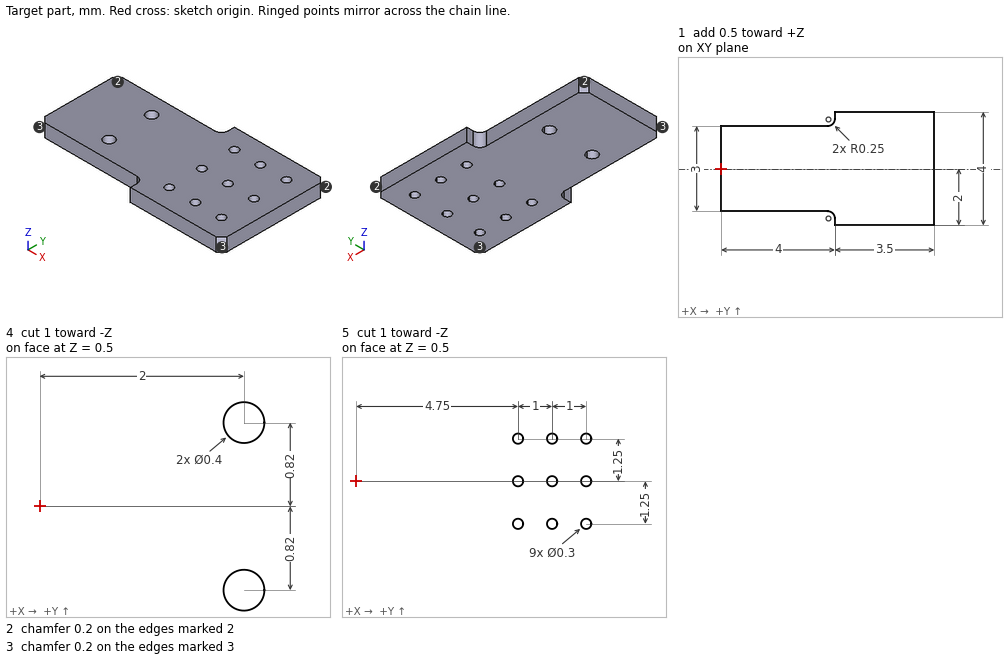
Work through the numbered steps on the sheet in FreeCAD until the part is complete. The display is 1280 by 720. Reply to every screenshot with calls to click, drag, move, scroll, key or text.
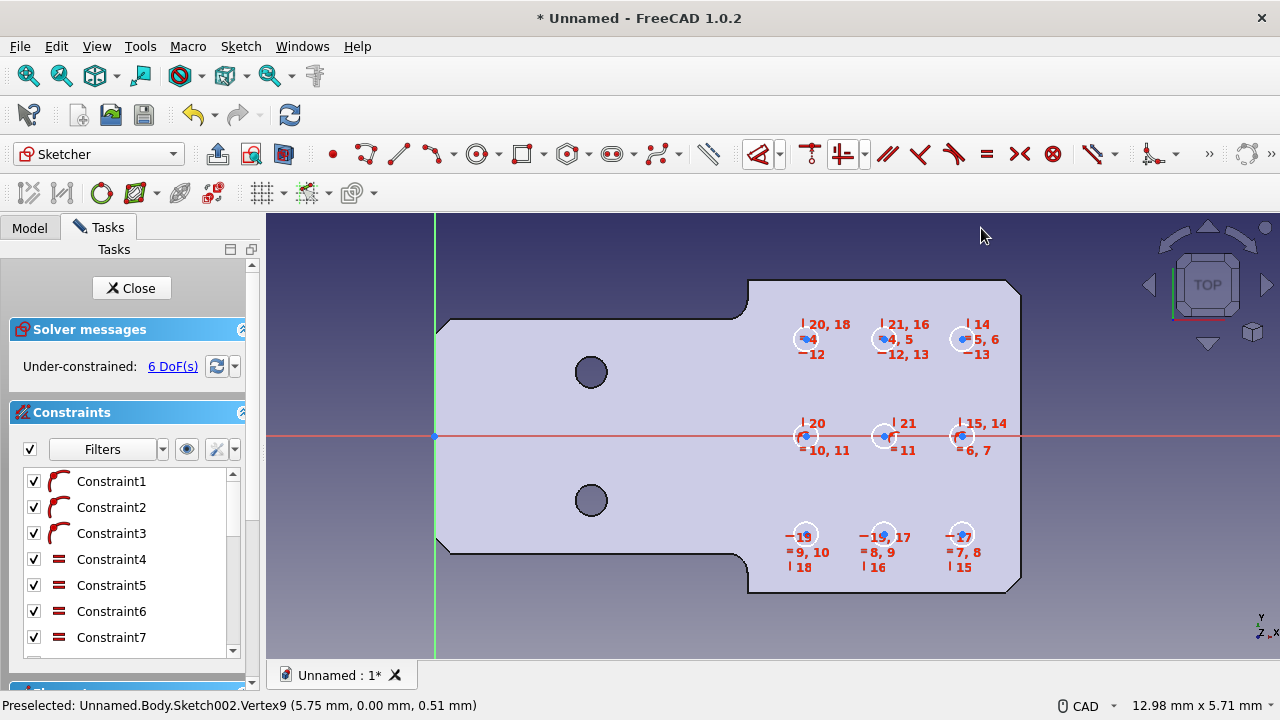
key(d)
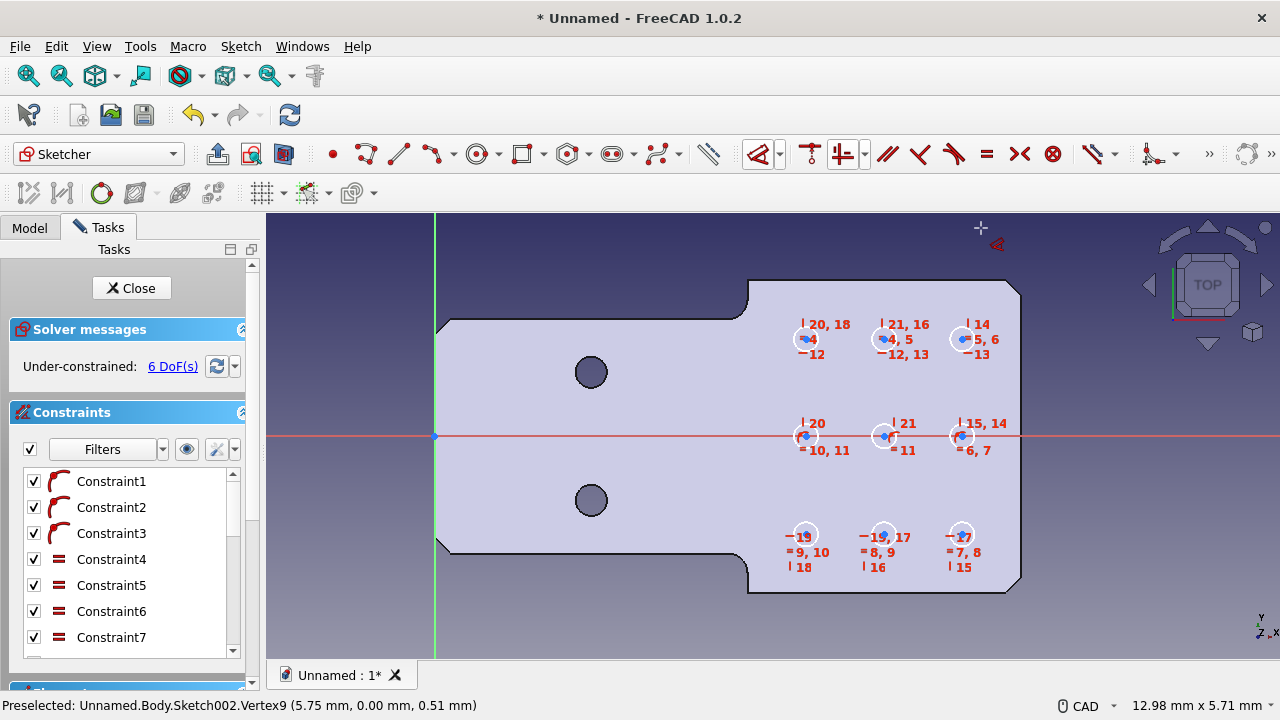
scroll(815, 331, up, 3)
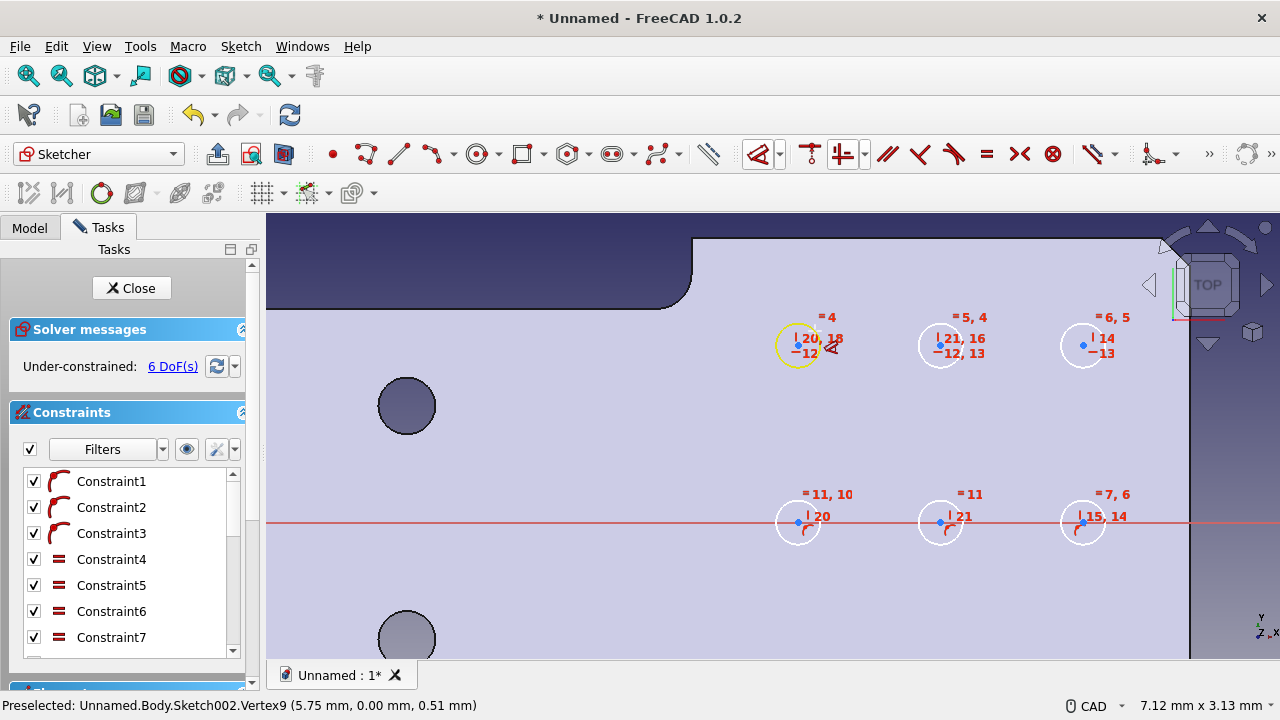
click(814, 330)
click(837, 308)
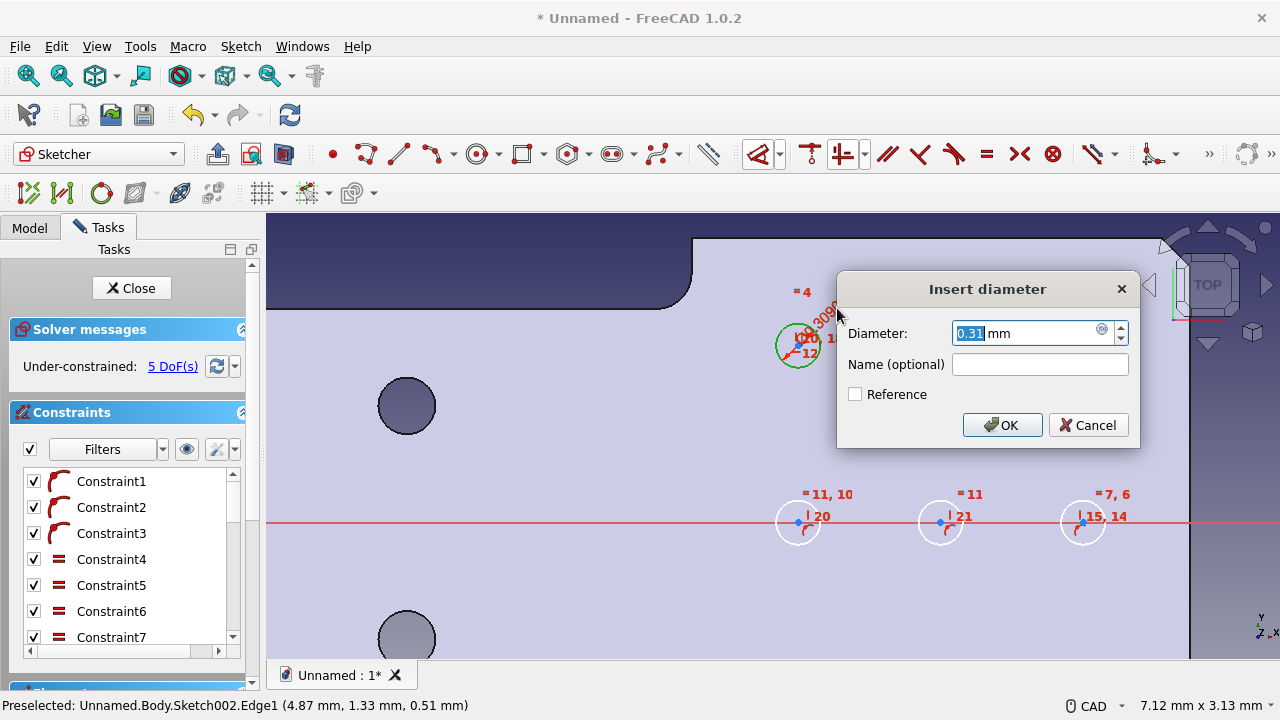
text(0.3)
key(Return)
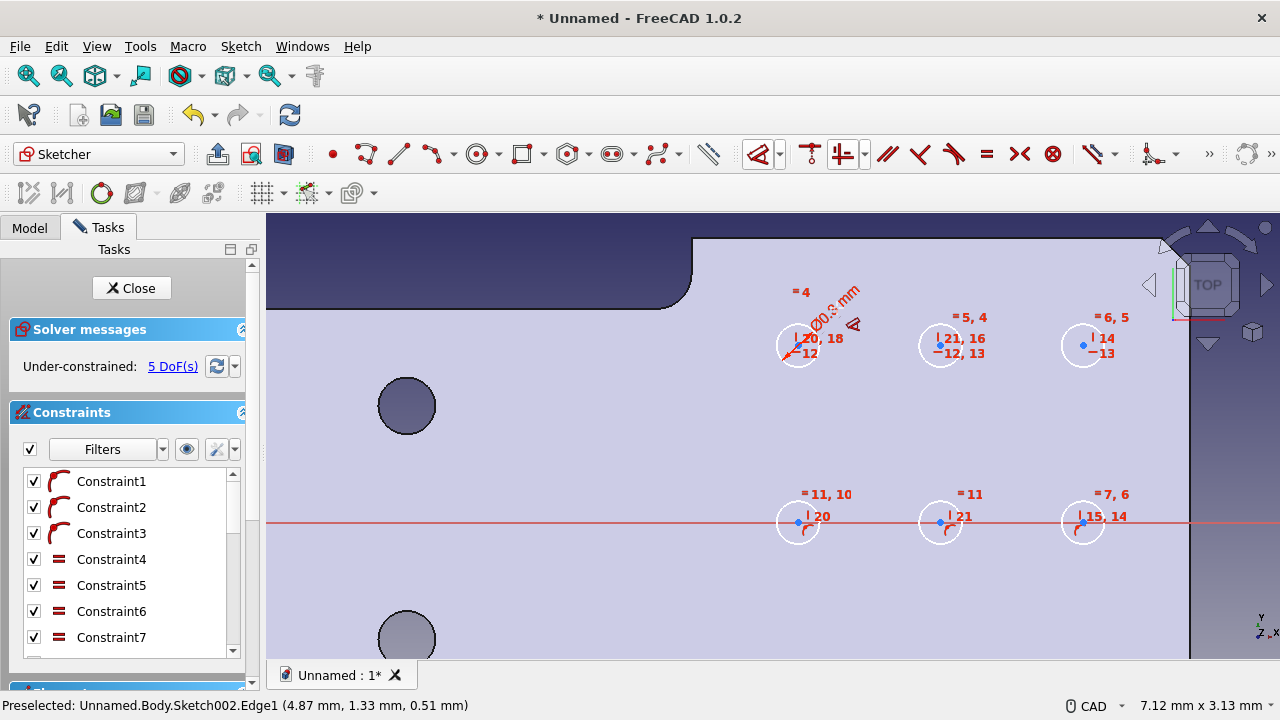
click(798, 346)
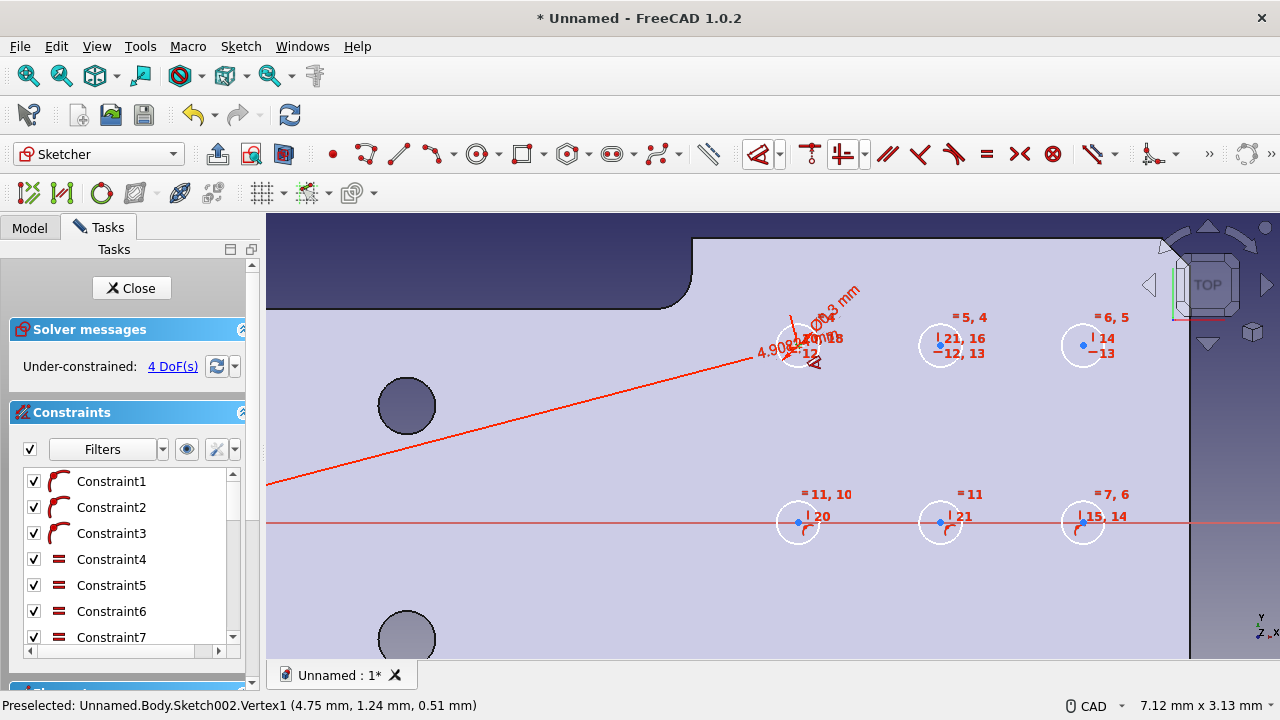
click(941, 346)
click(919, 312)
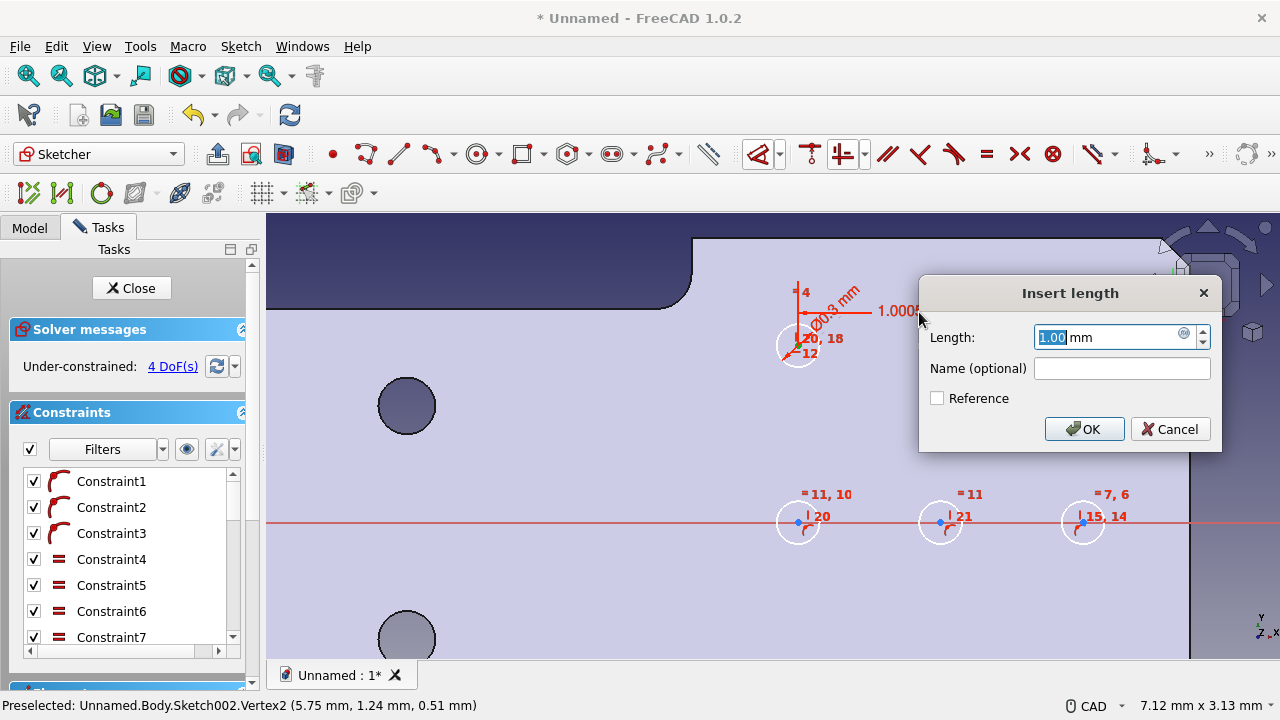
text(1)
key(Return)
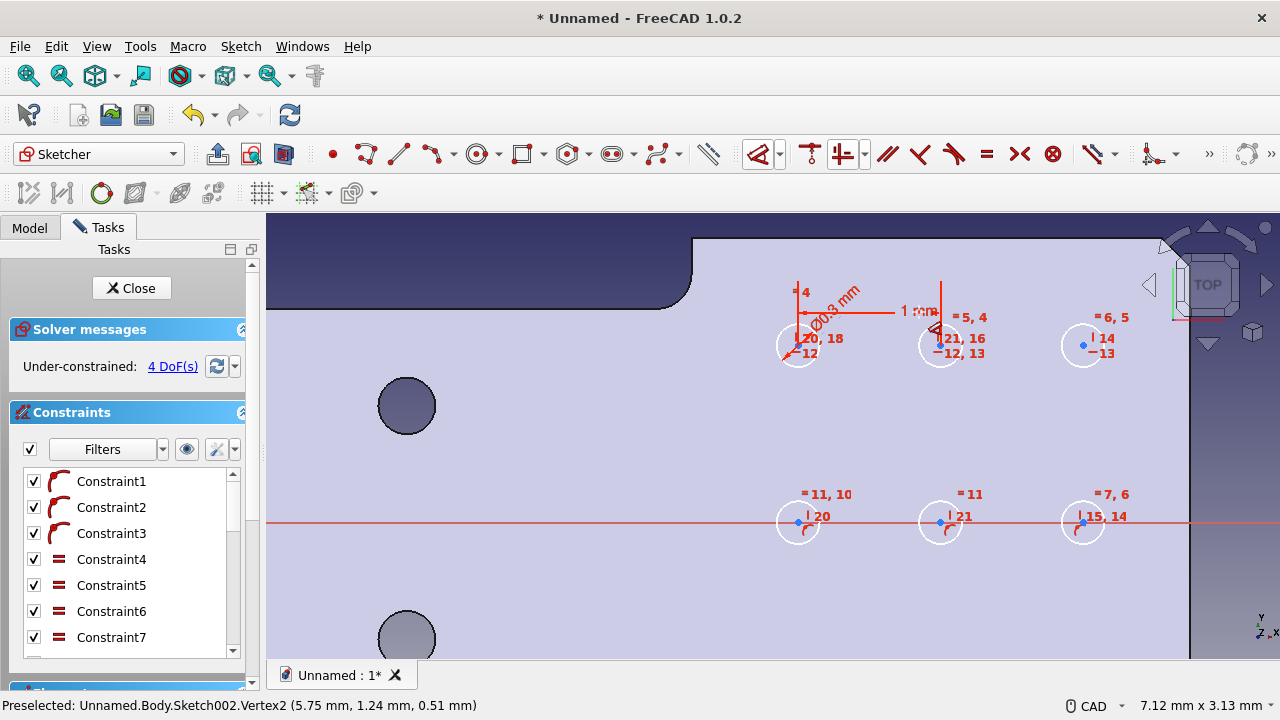
click(941, 346)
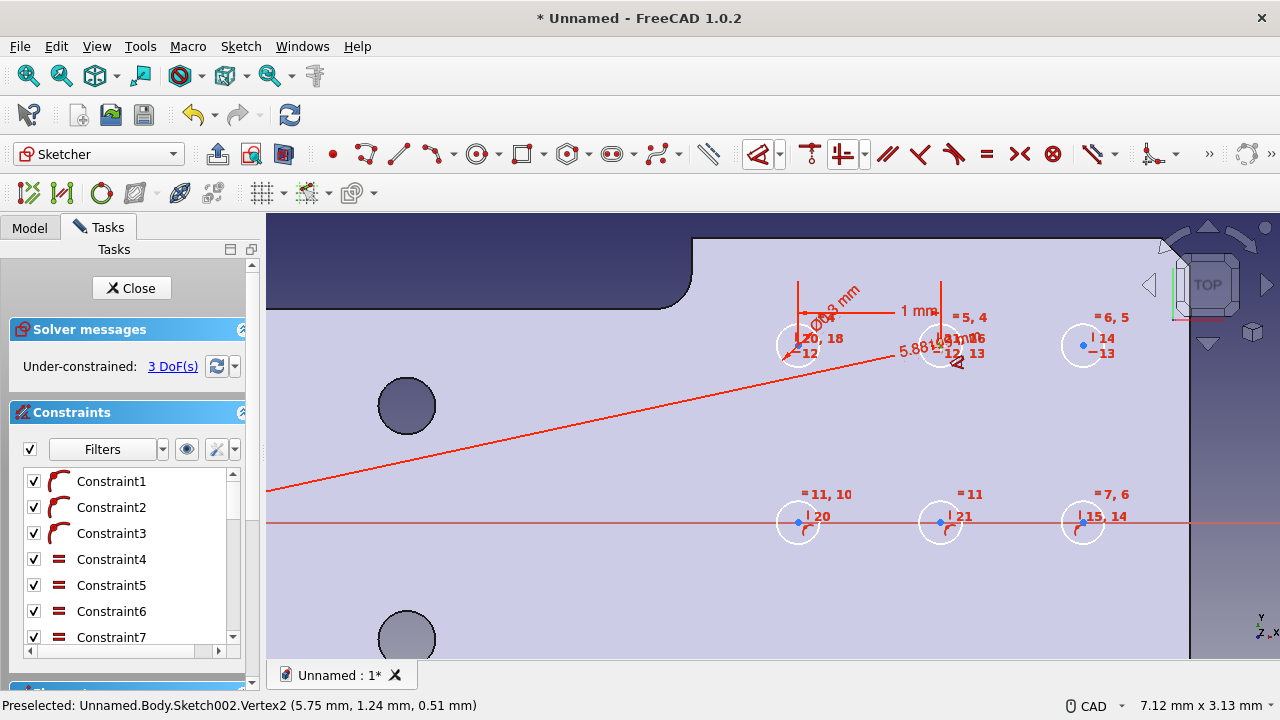
click(1083, 346)
click(1012, 312)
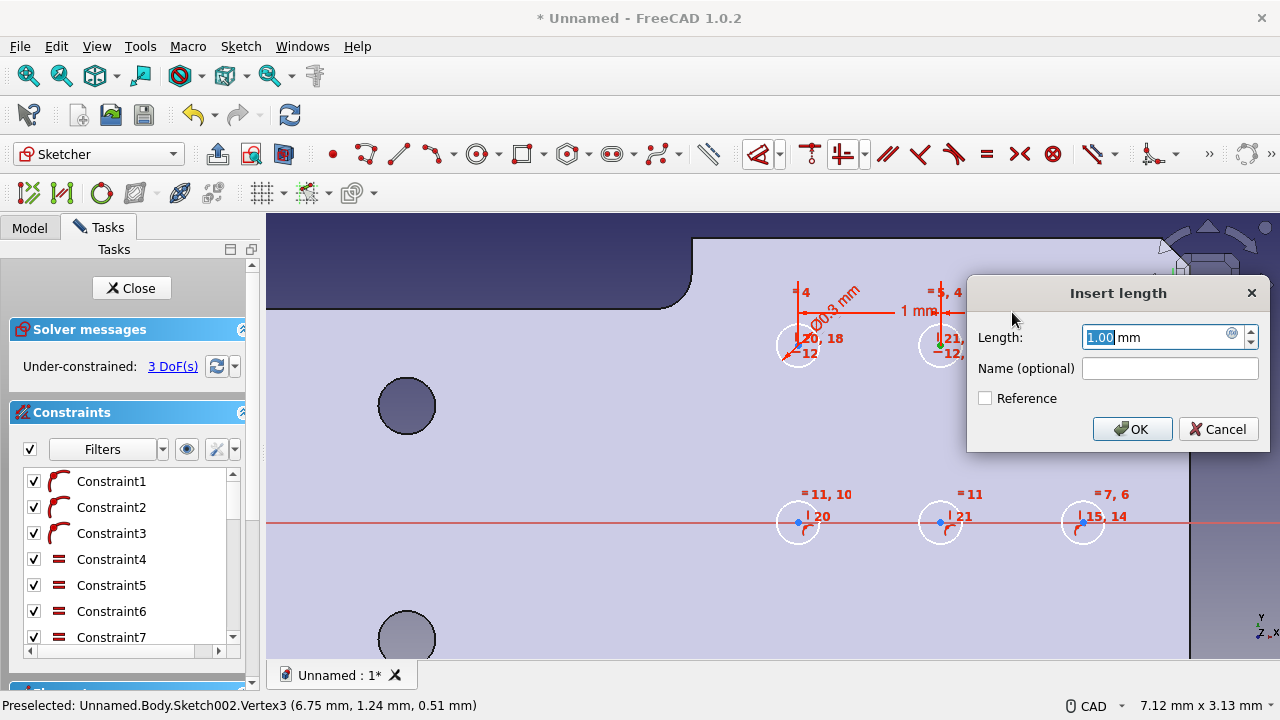
text(1)
key(Return)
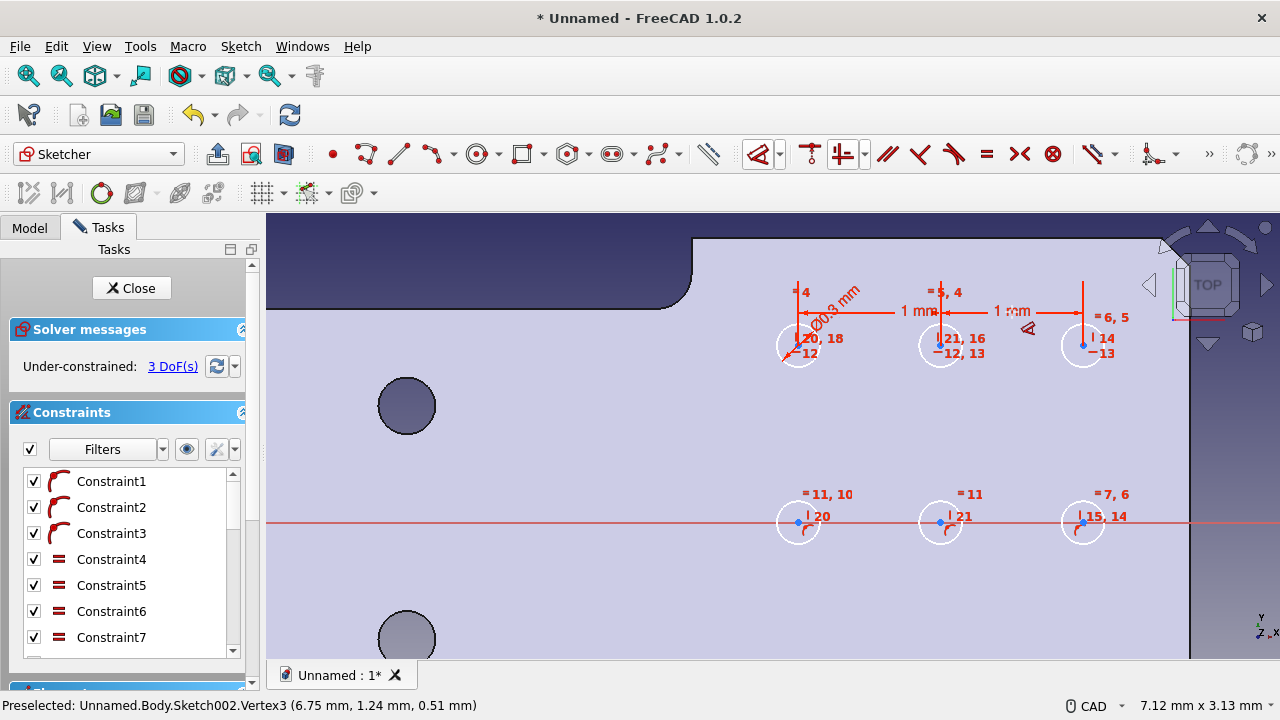
click(798, 346)
click(546, 312)